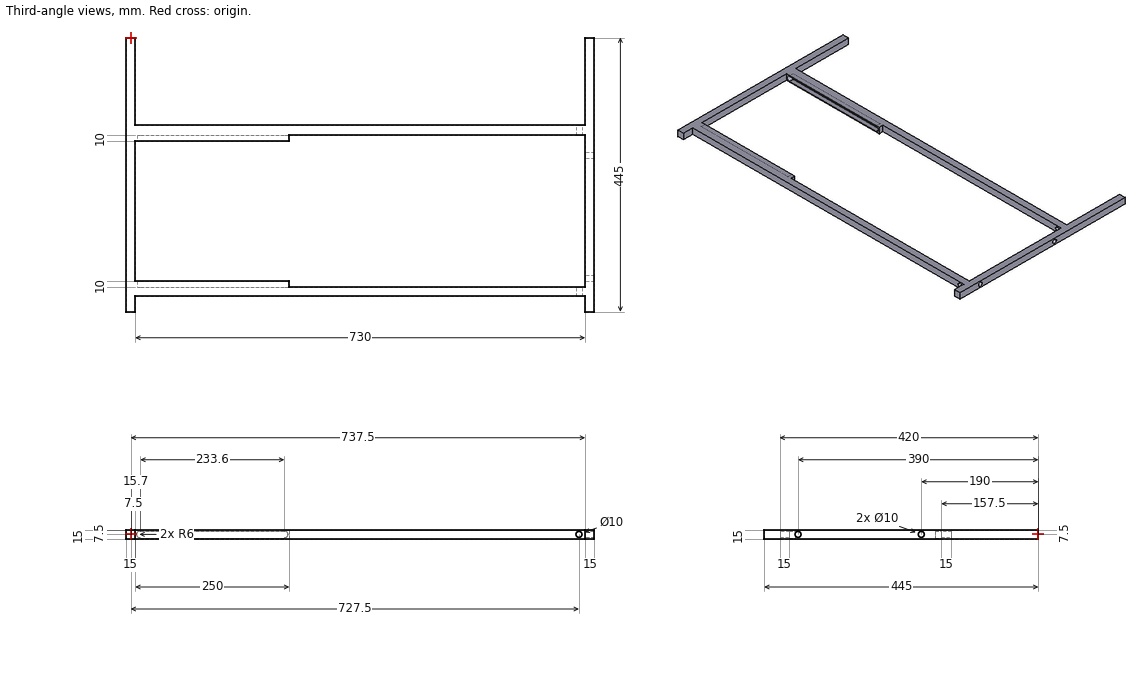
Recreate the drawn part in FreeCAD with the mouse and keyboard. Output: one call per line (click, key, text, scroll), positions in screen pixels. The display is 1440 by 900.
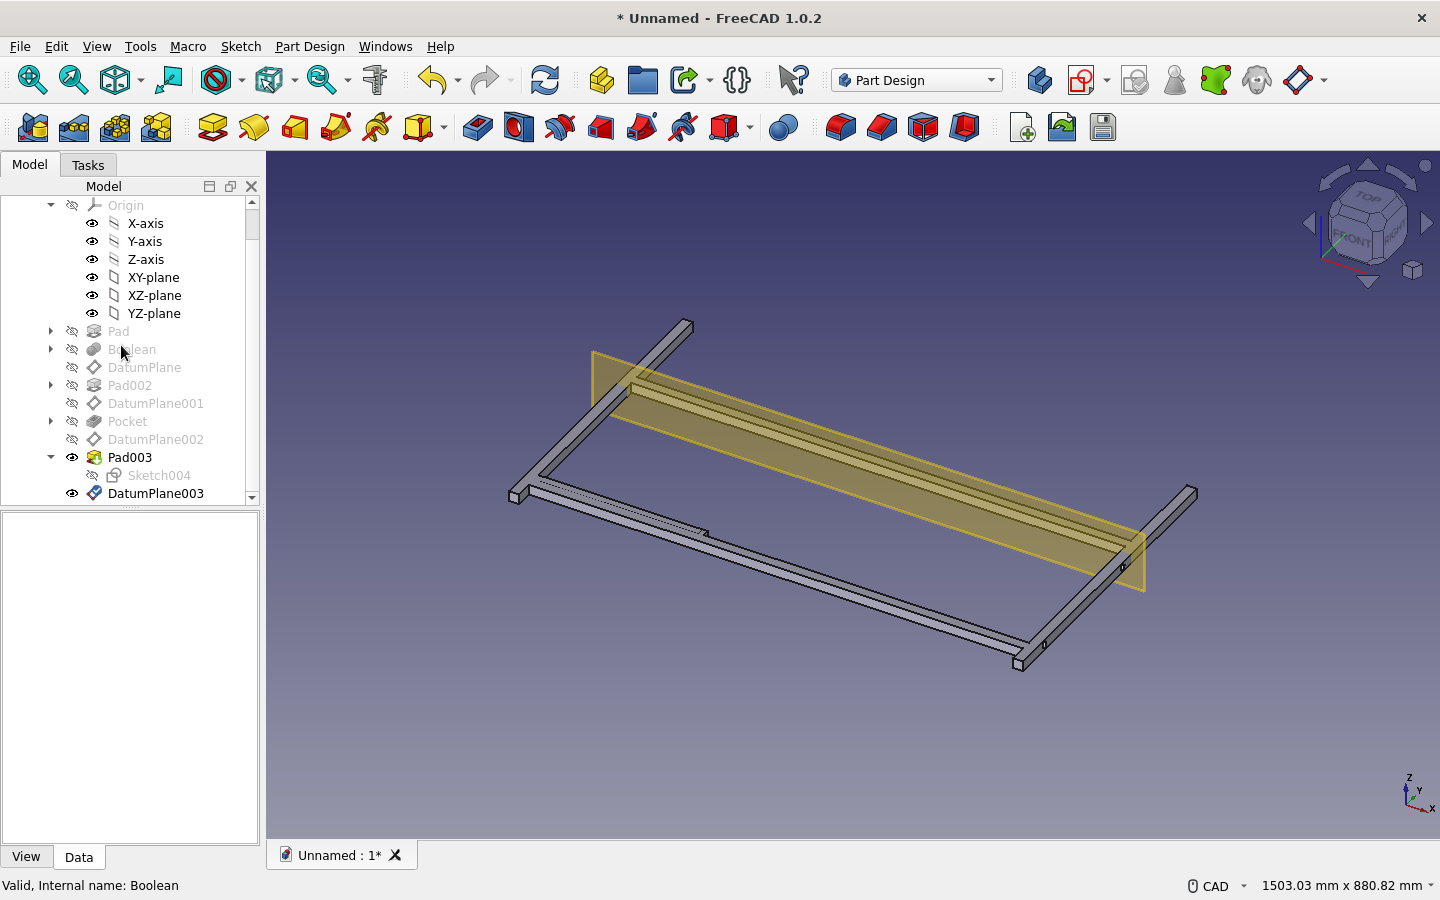
click(117, 493)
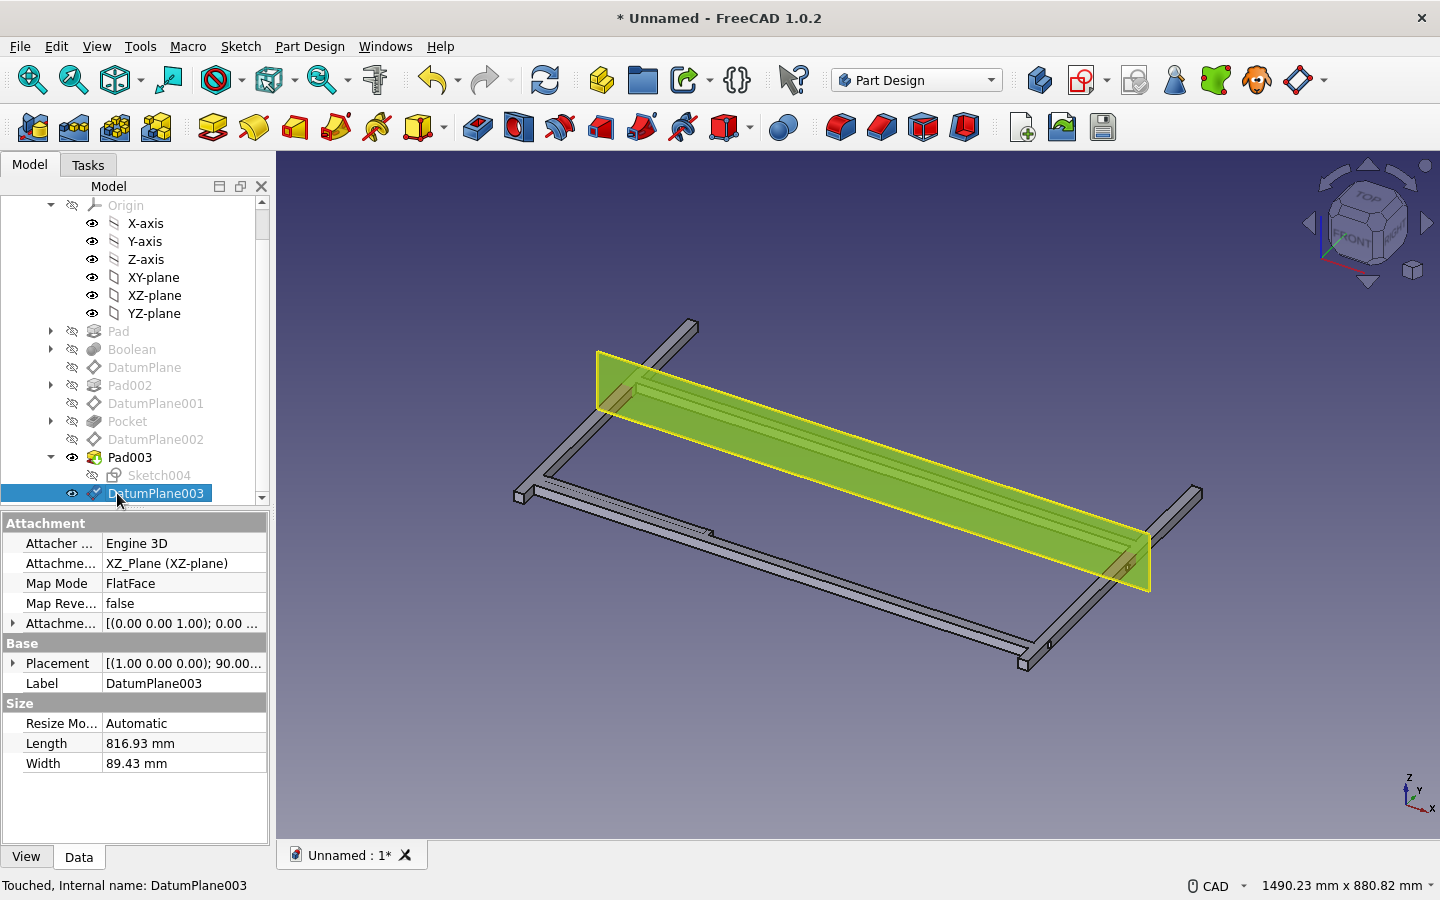
click(1080, 80)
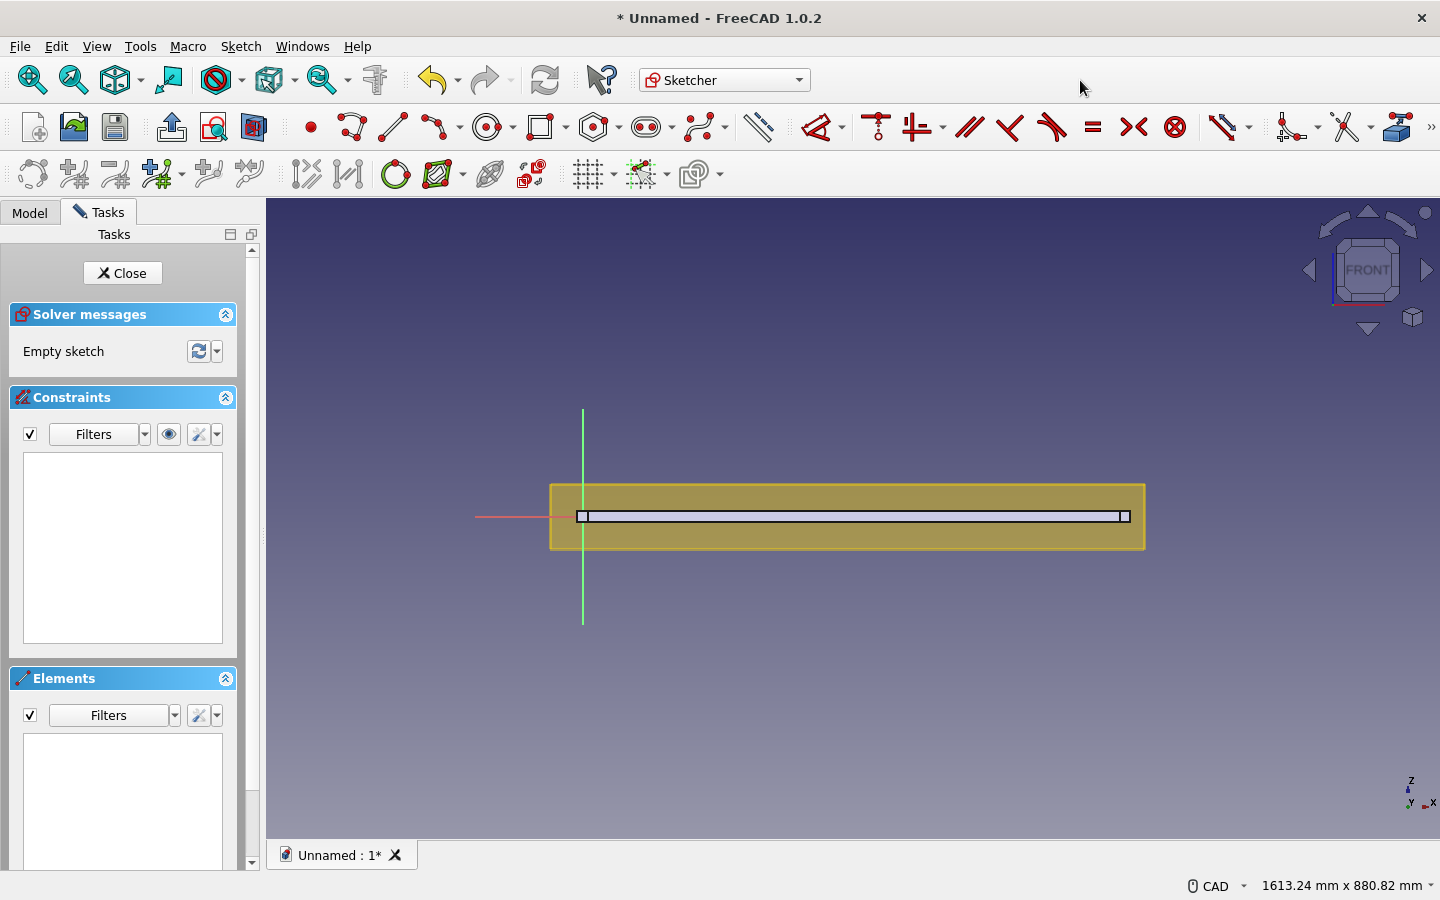
click(254, 128)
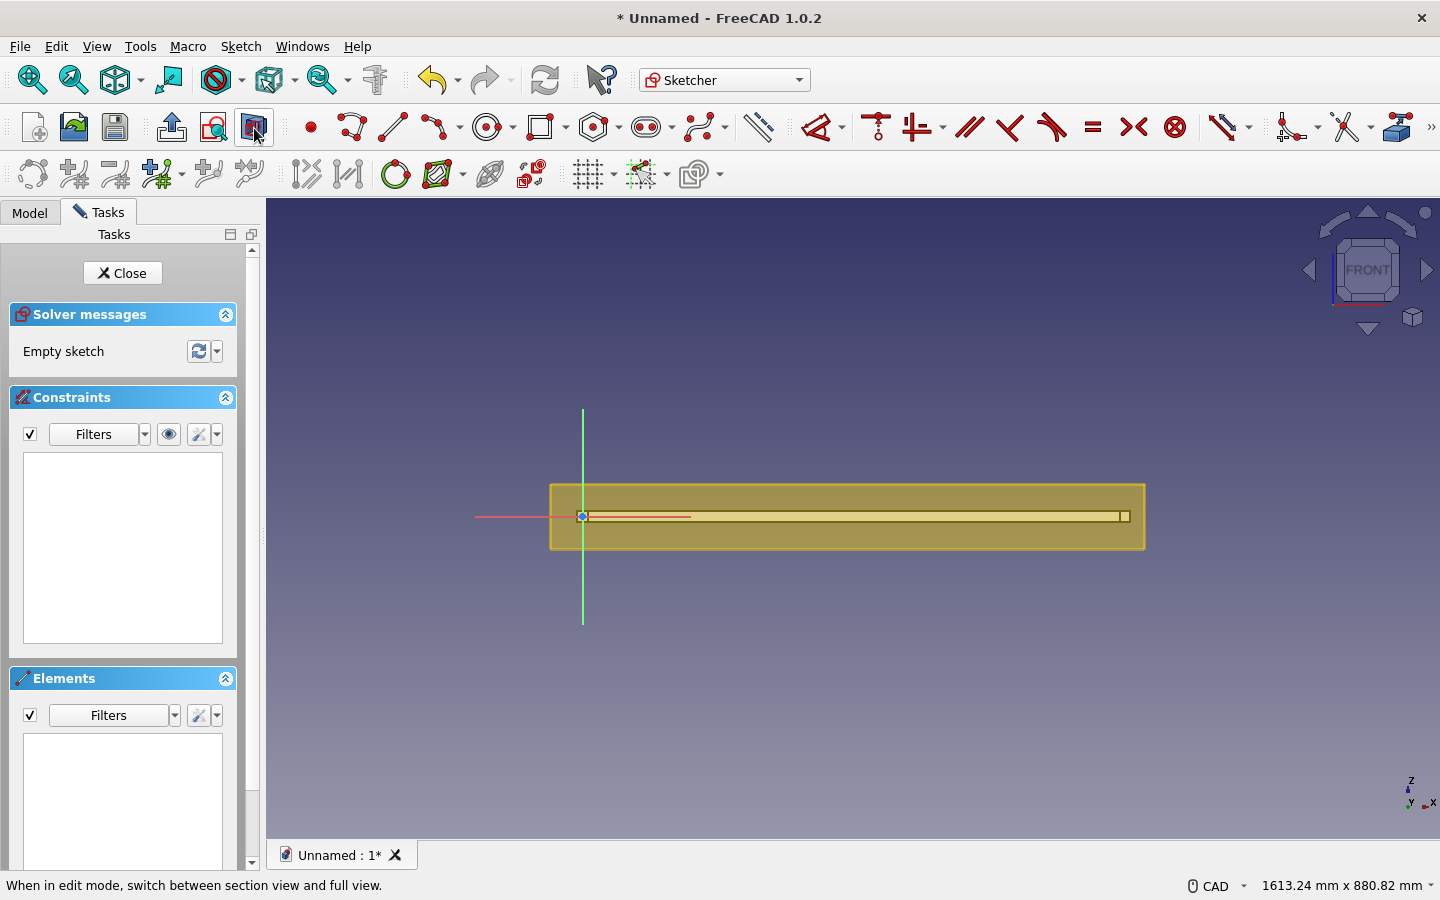
scroll(641, 516, up, 7)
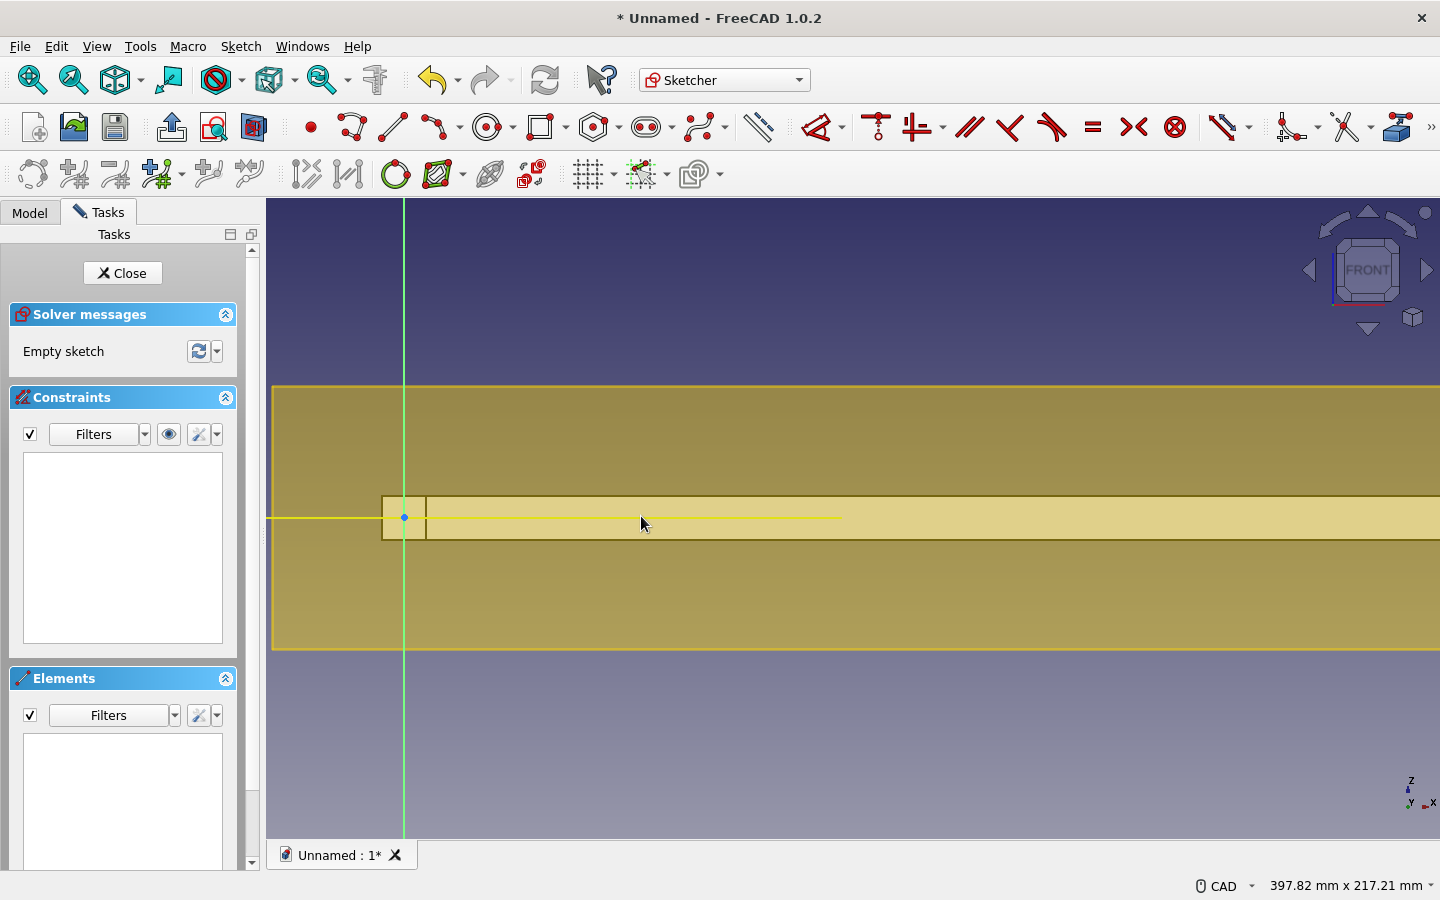
click(540, 128)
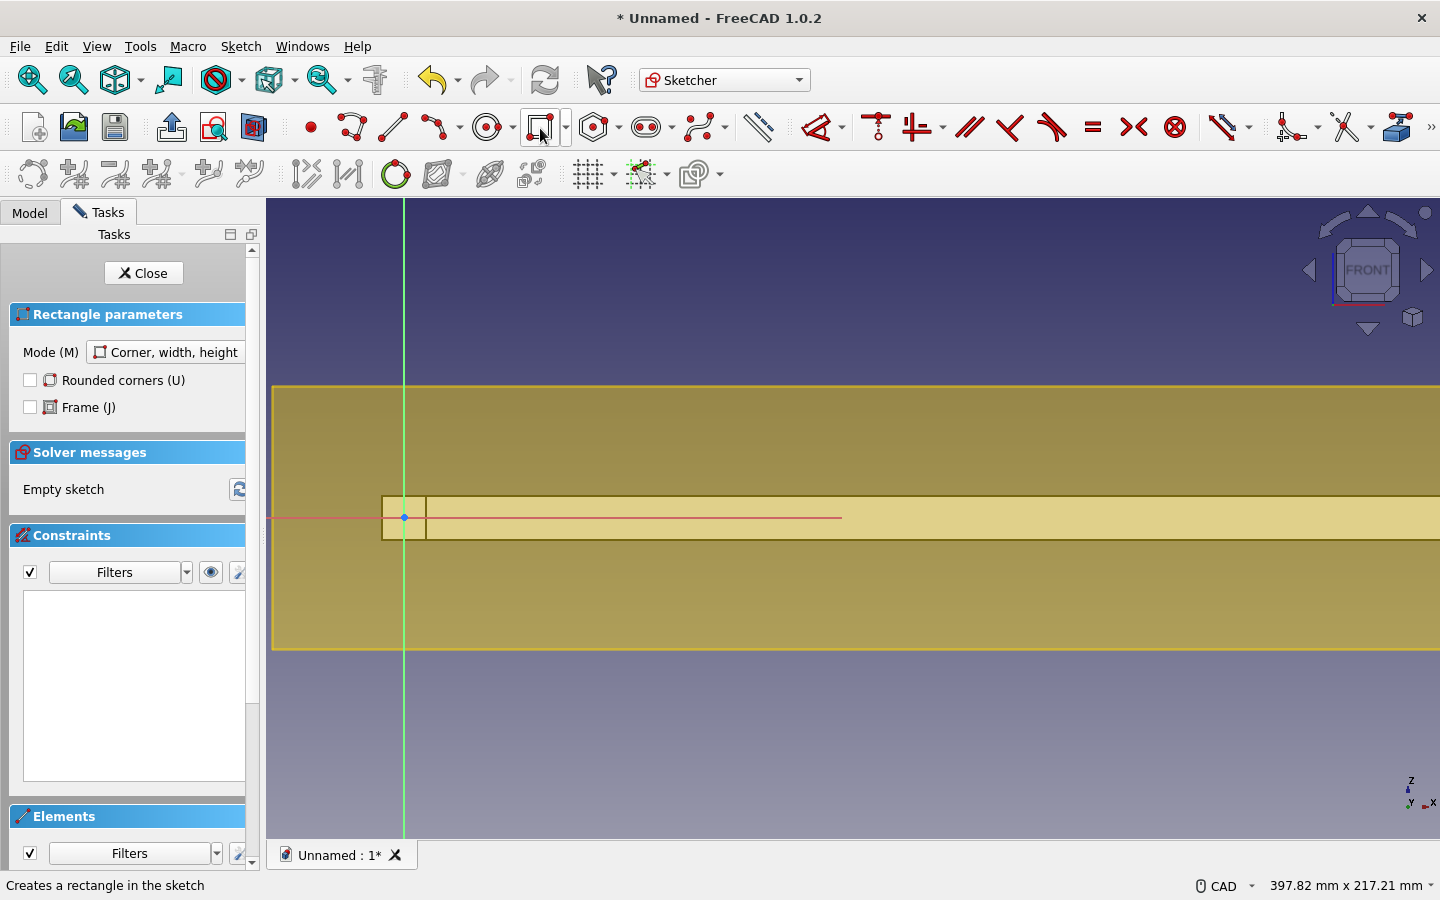
click(426, 496)
click(1164, 540)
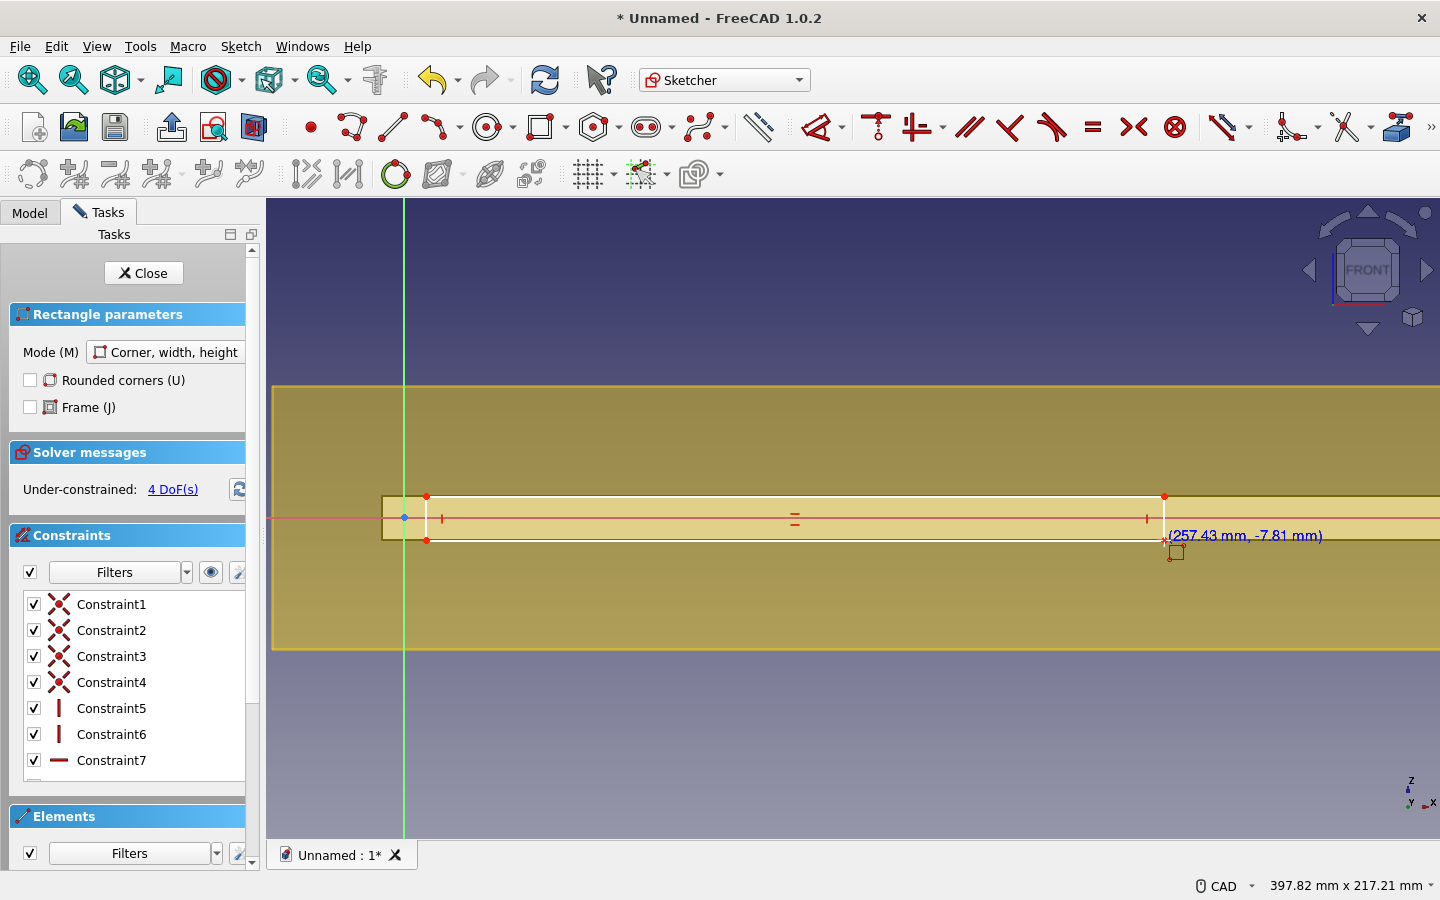
click(646, 128)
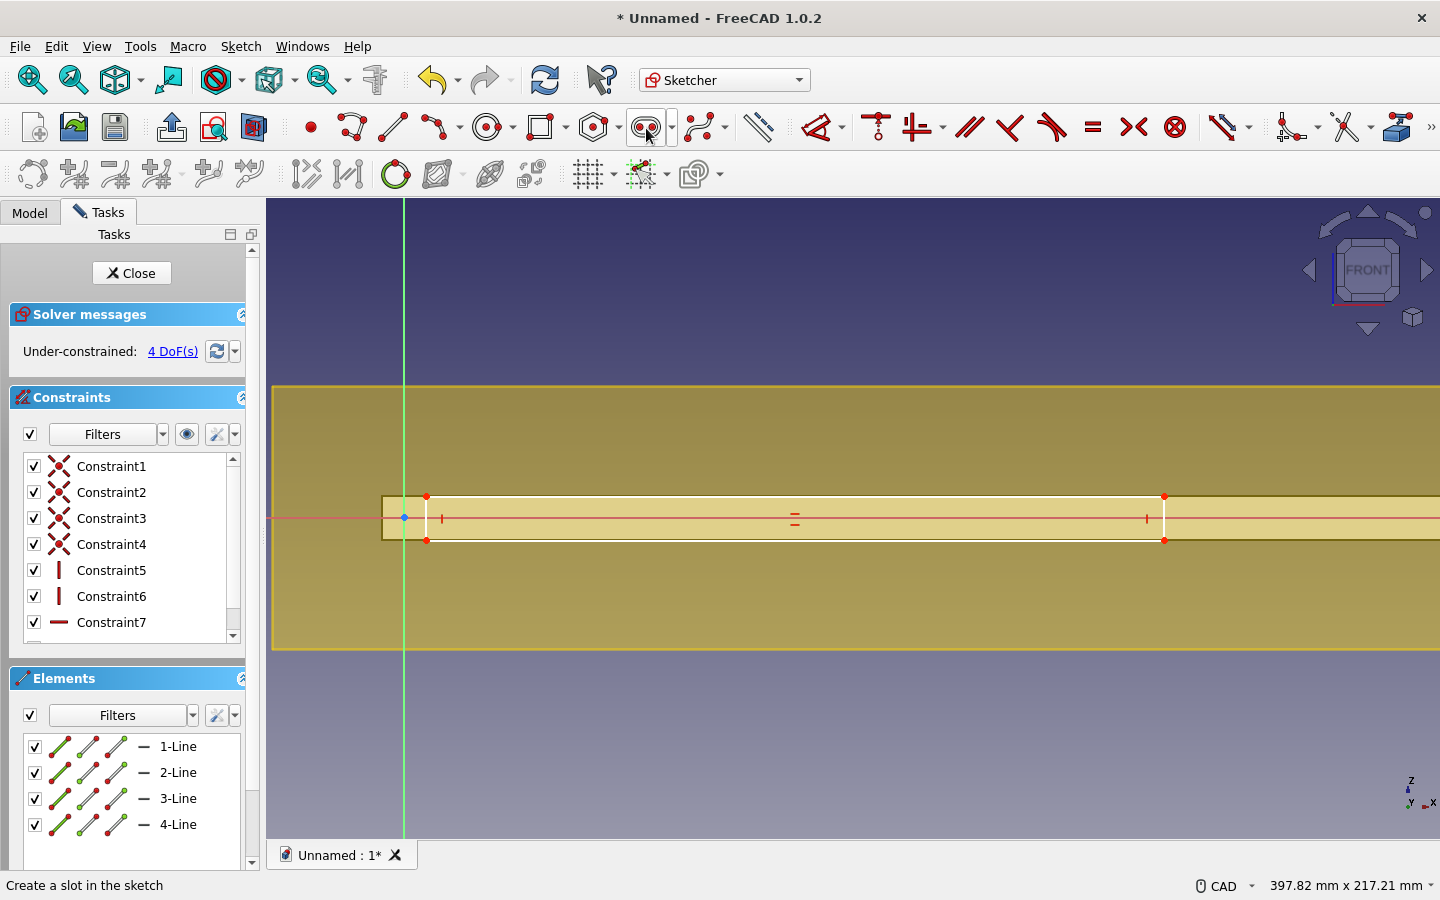
scroll(451, 518, up, 2)